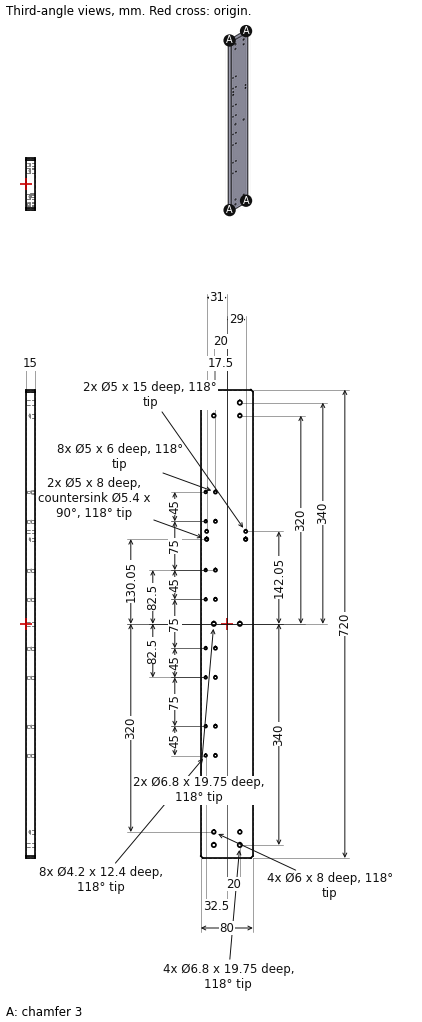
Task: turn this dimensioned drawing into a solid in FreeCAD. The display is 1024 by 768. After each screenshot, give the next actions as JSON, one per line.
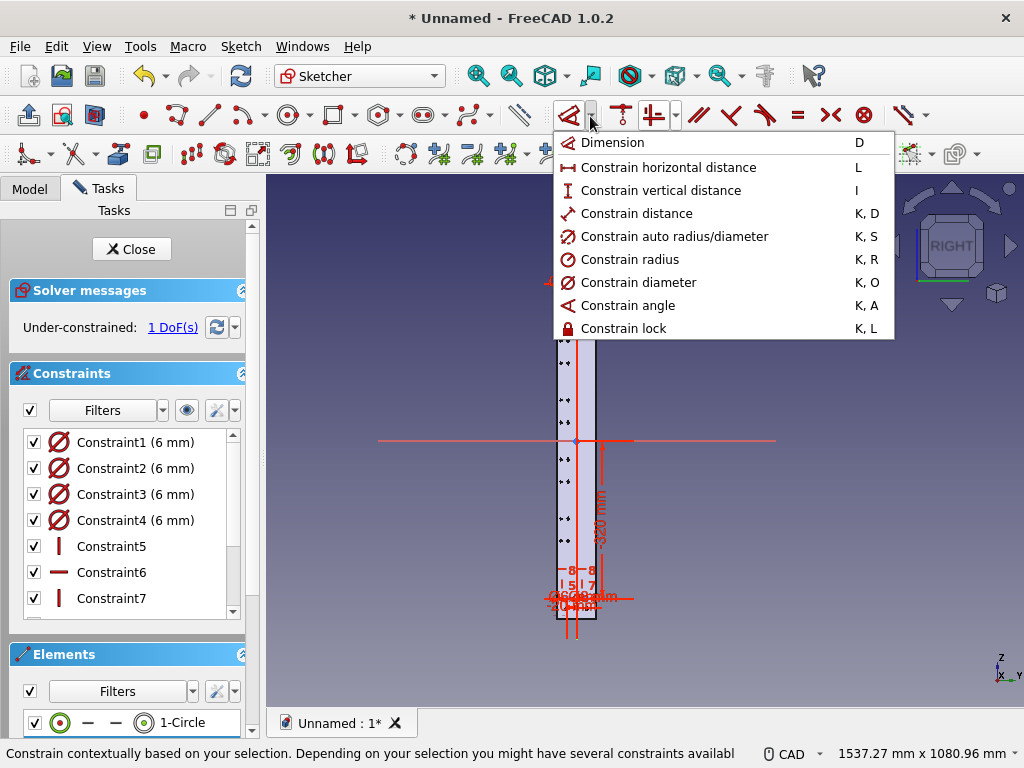
{"action": "left_click", "coordinate": [724, 190]}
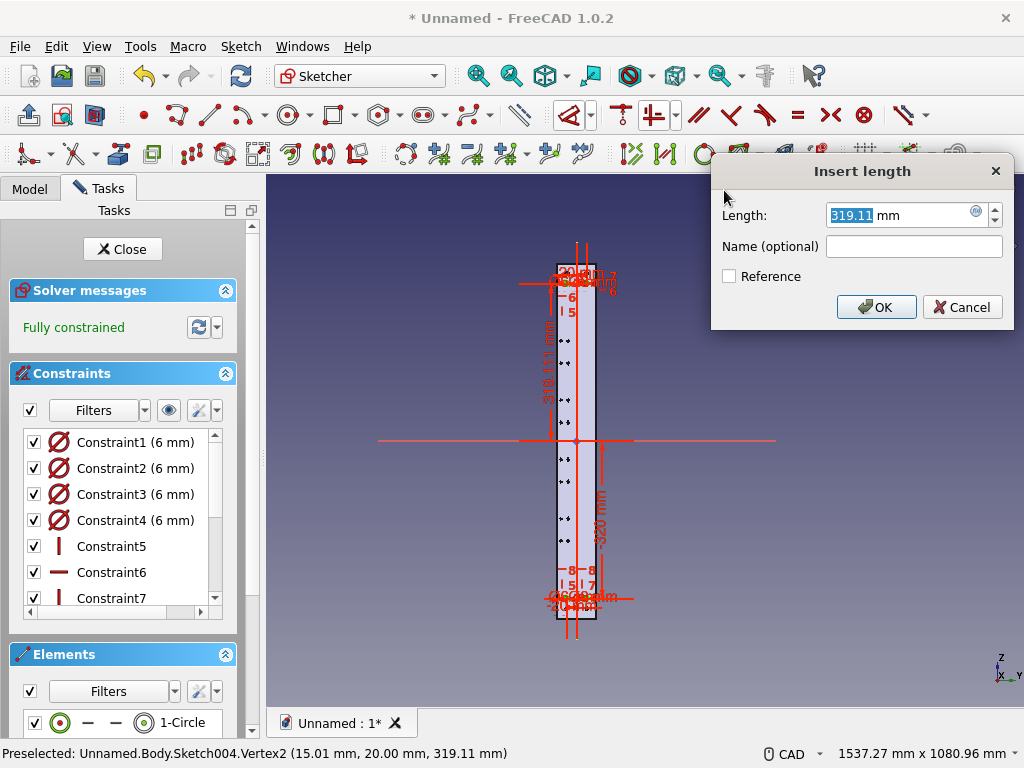
{"action": "type", "text": "320"}
{"action": "key", "text": "Return"}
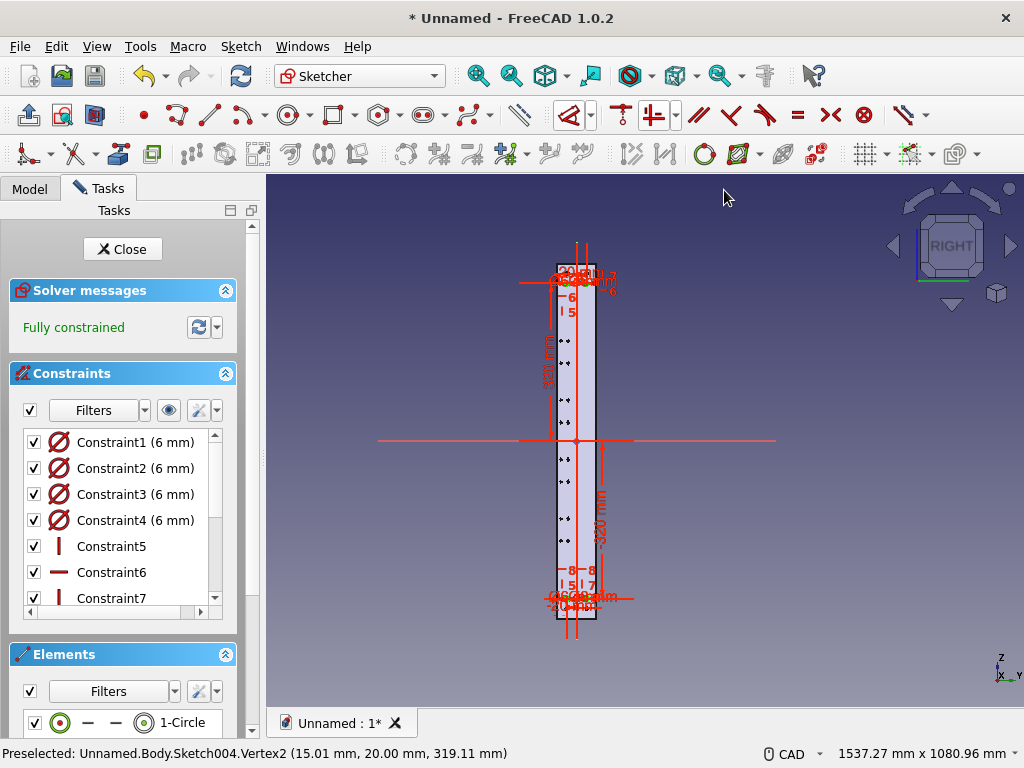
{"action": "left_click", "coordinate": [123, 249]}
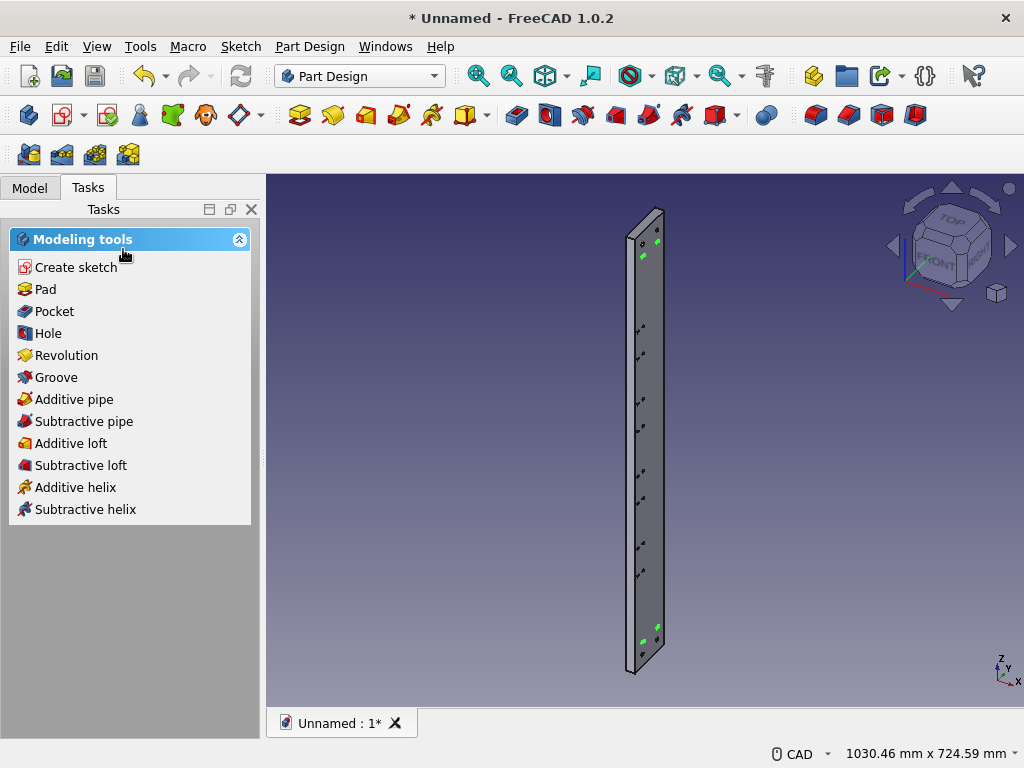
{"action": "left_click", "coordinate": [550, 116]}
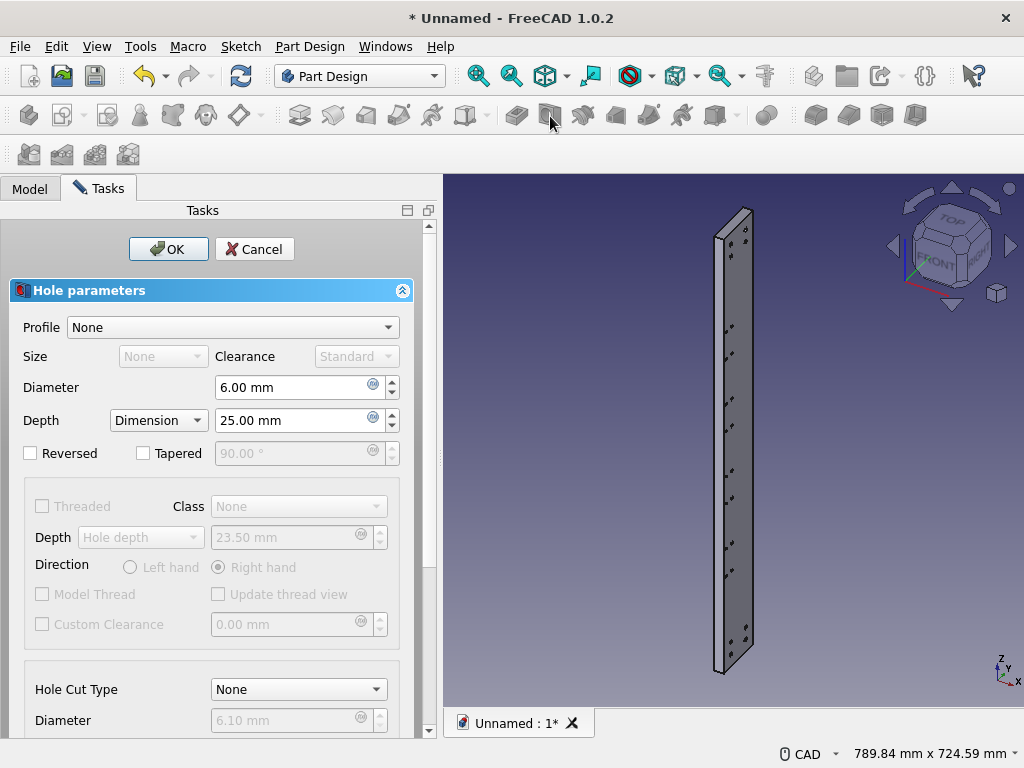
{"action": "triple_click", "coordinate": [300, 388]}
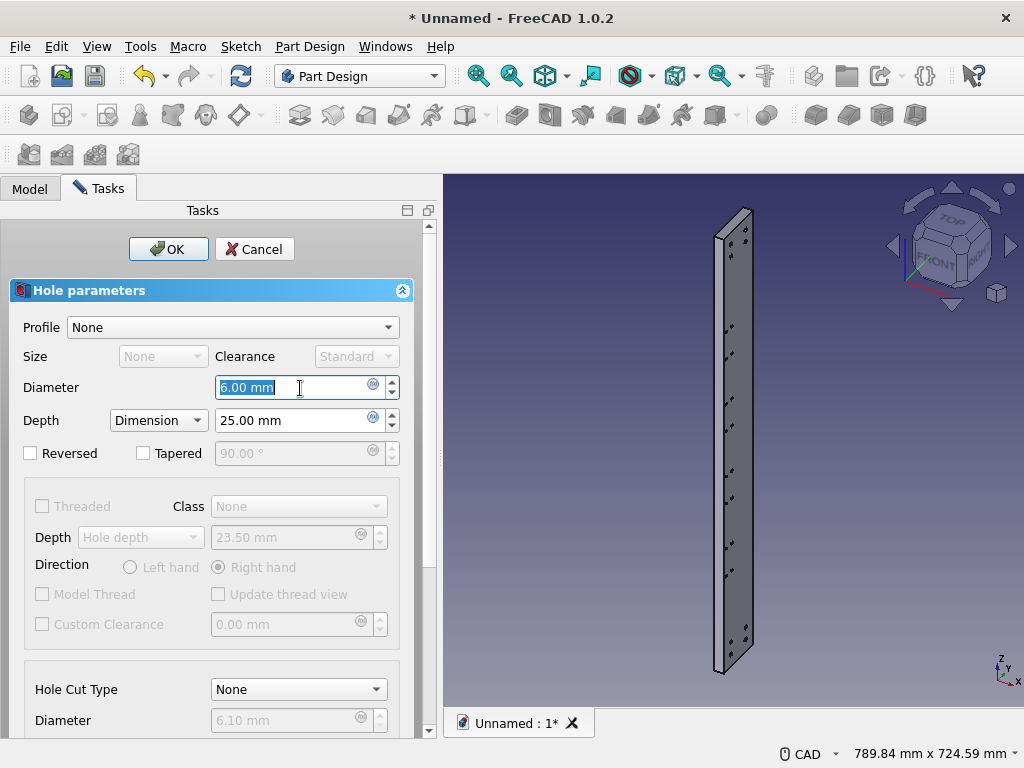
{"action": "type", "text": "6"}
{"action": "key", "text": "Tab"}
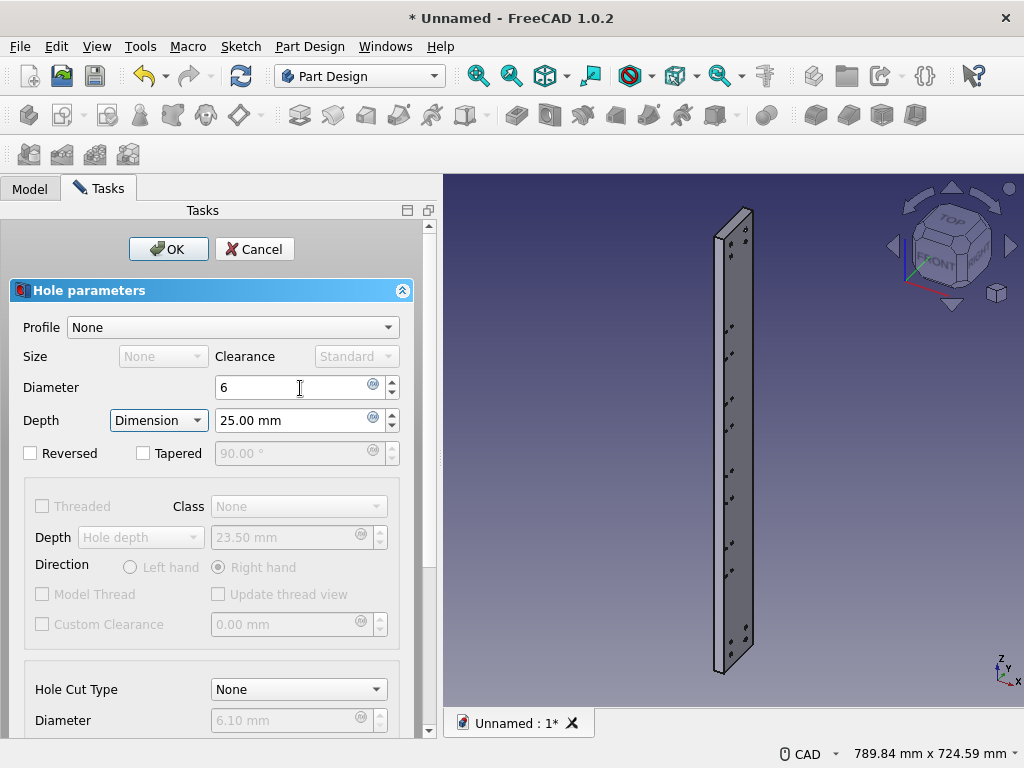
{"action": "triple_click", "coordinate": [300, 420]}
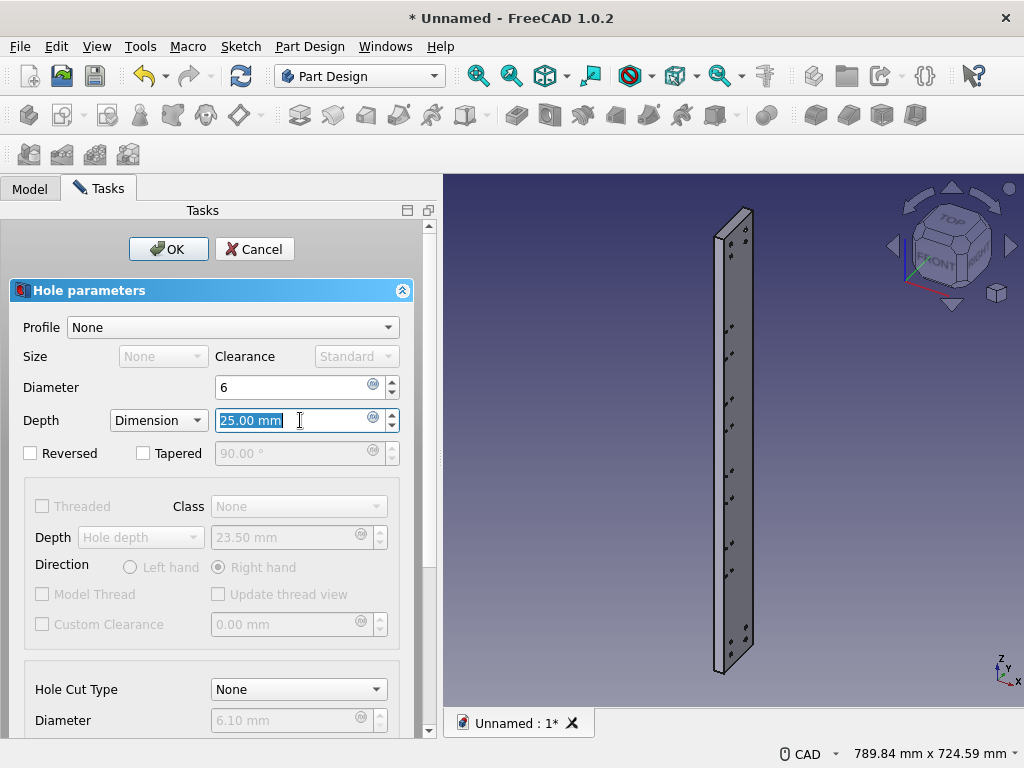
{"action": "type", "text": "8"}
{"action": "key", "text": "Tab"}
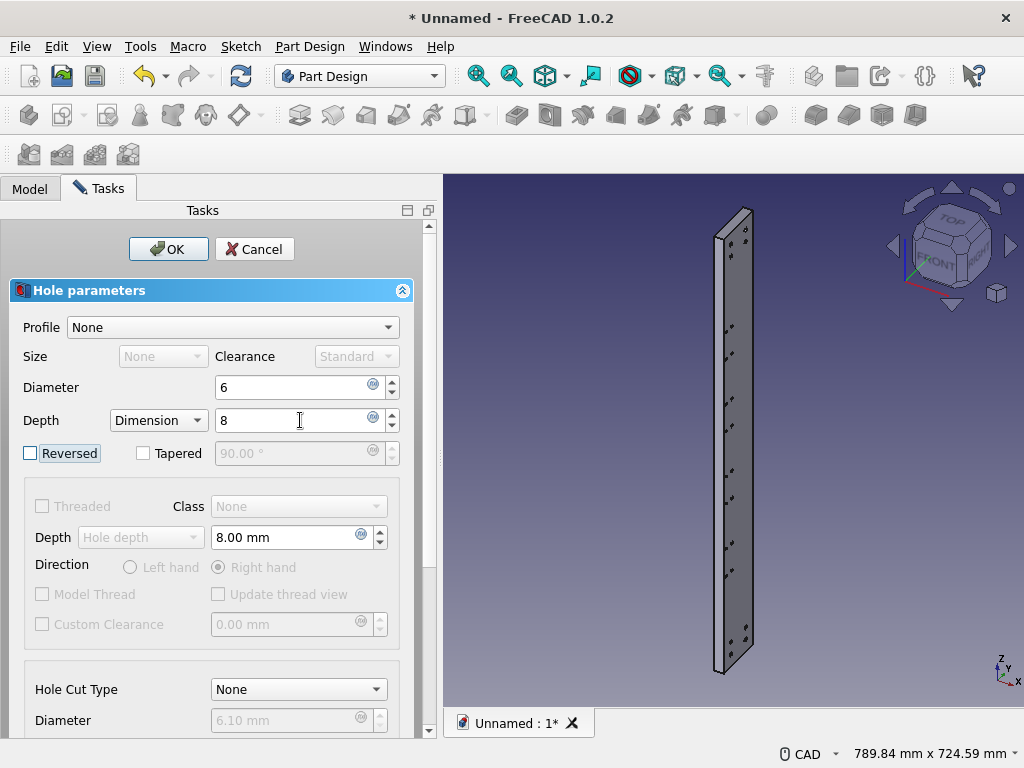
{"action": "left_click", "coordinate": [169, 249]}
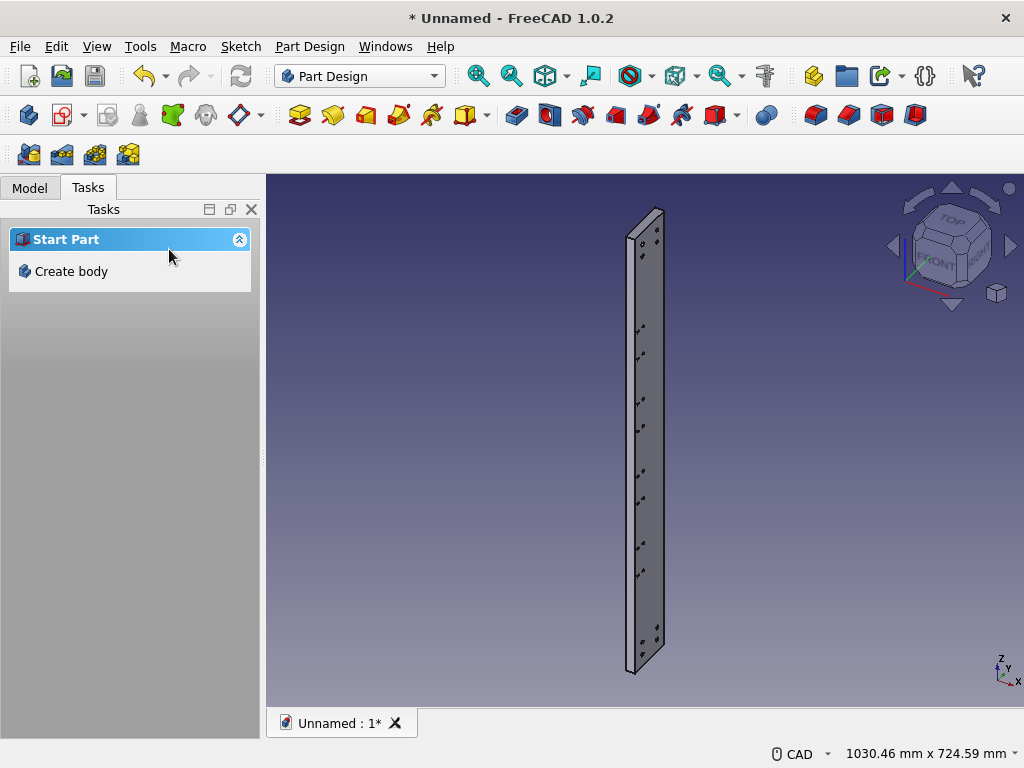
{"action": "left_click", "coordinate": [650, 441]}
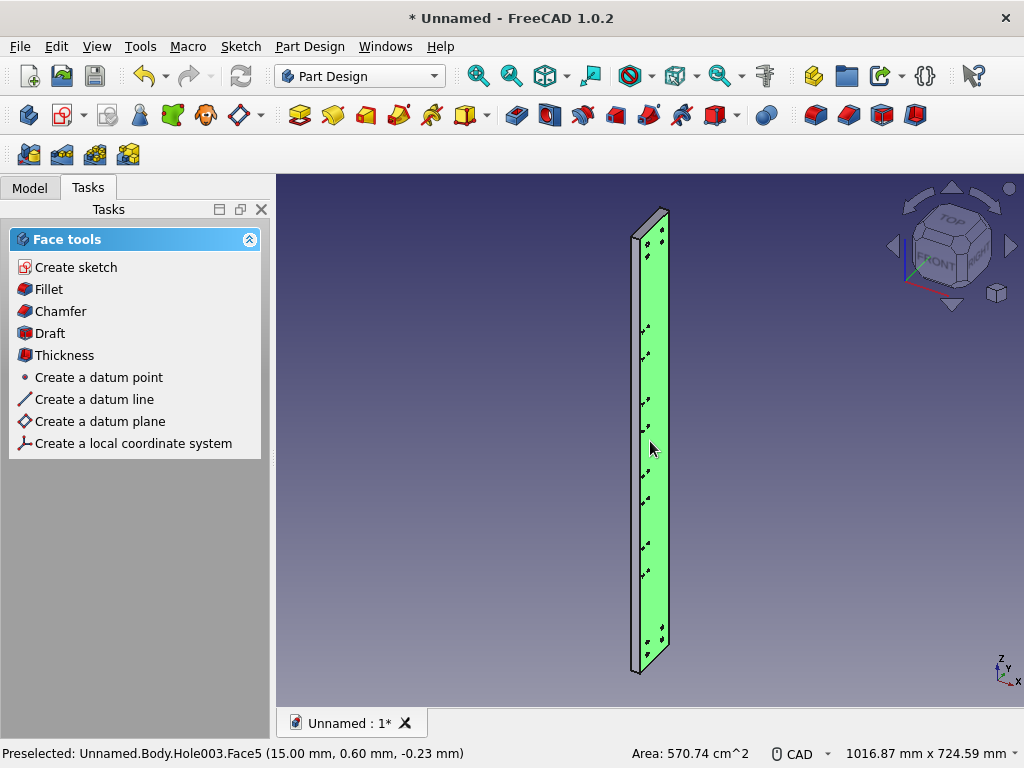
{"action": "left_click", "coordinate": [62, 116]}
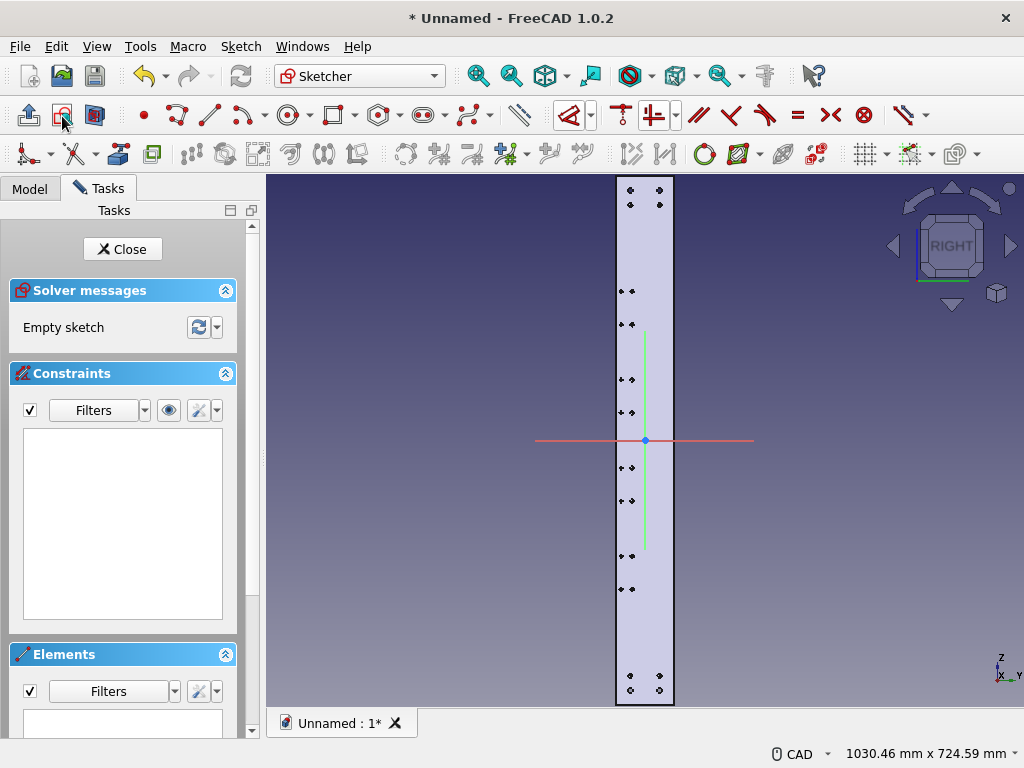
{"action": "scroll", "coordinate": [652, 440], "scroll_direction": "up", "scroll_amount": 12}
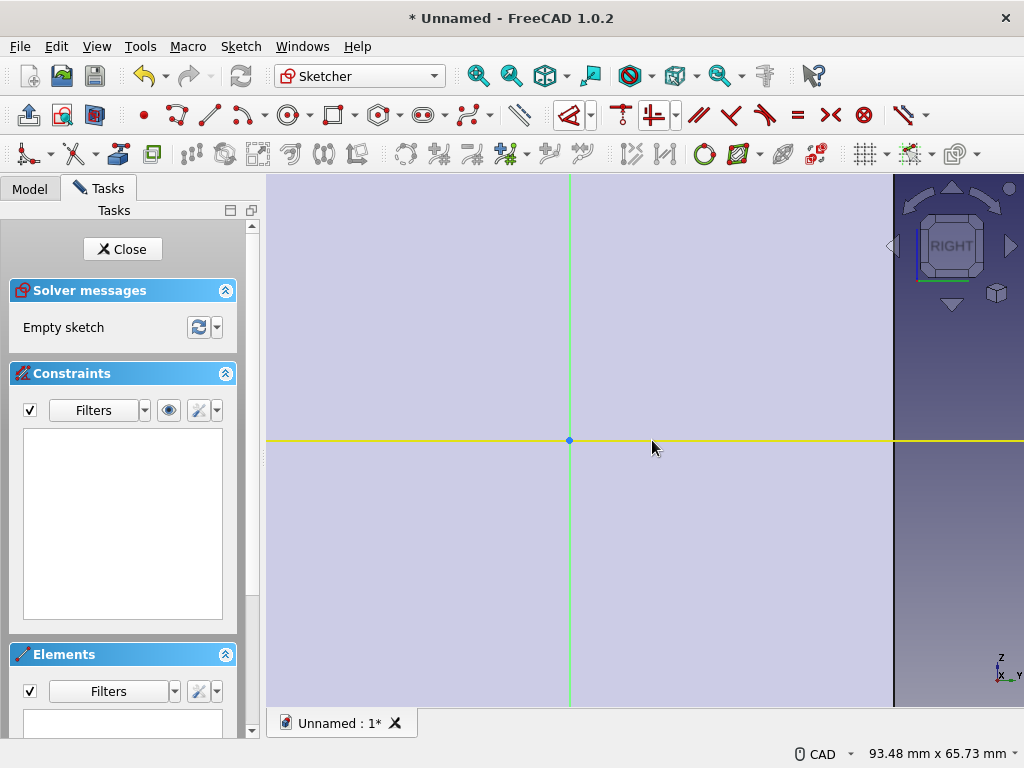
{"action": "key", "text": "g c"}